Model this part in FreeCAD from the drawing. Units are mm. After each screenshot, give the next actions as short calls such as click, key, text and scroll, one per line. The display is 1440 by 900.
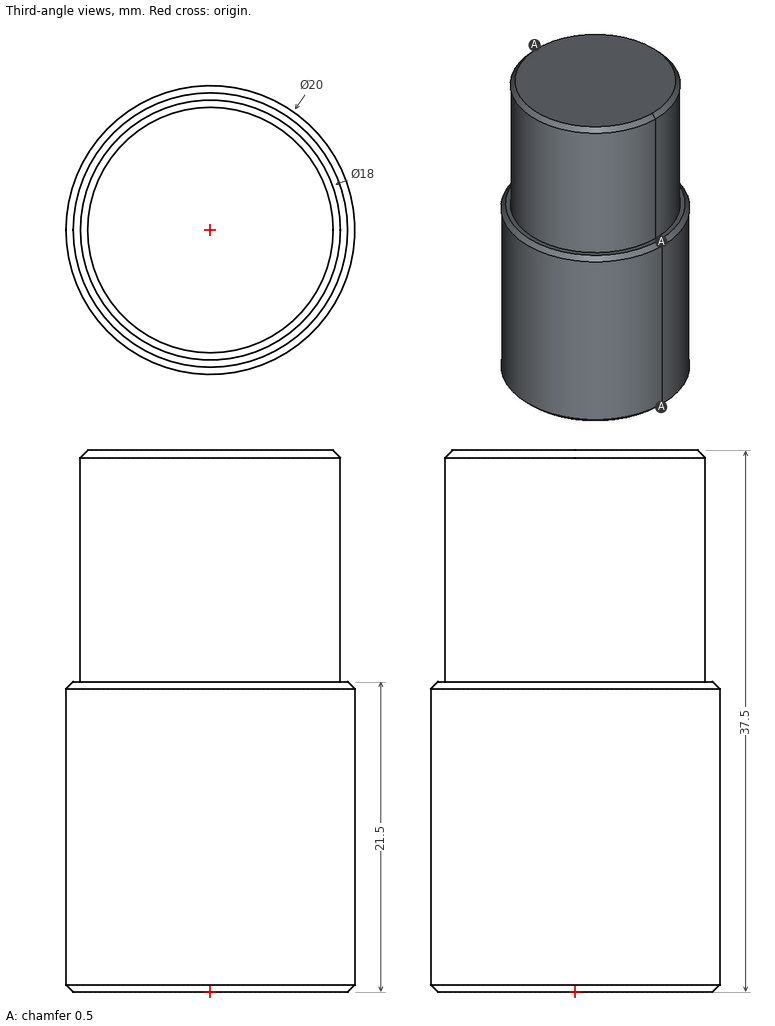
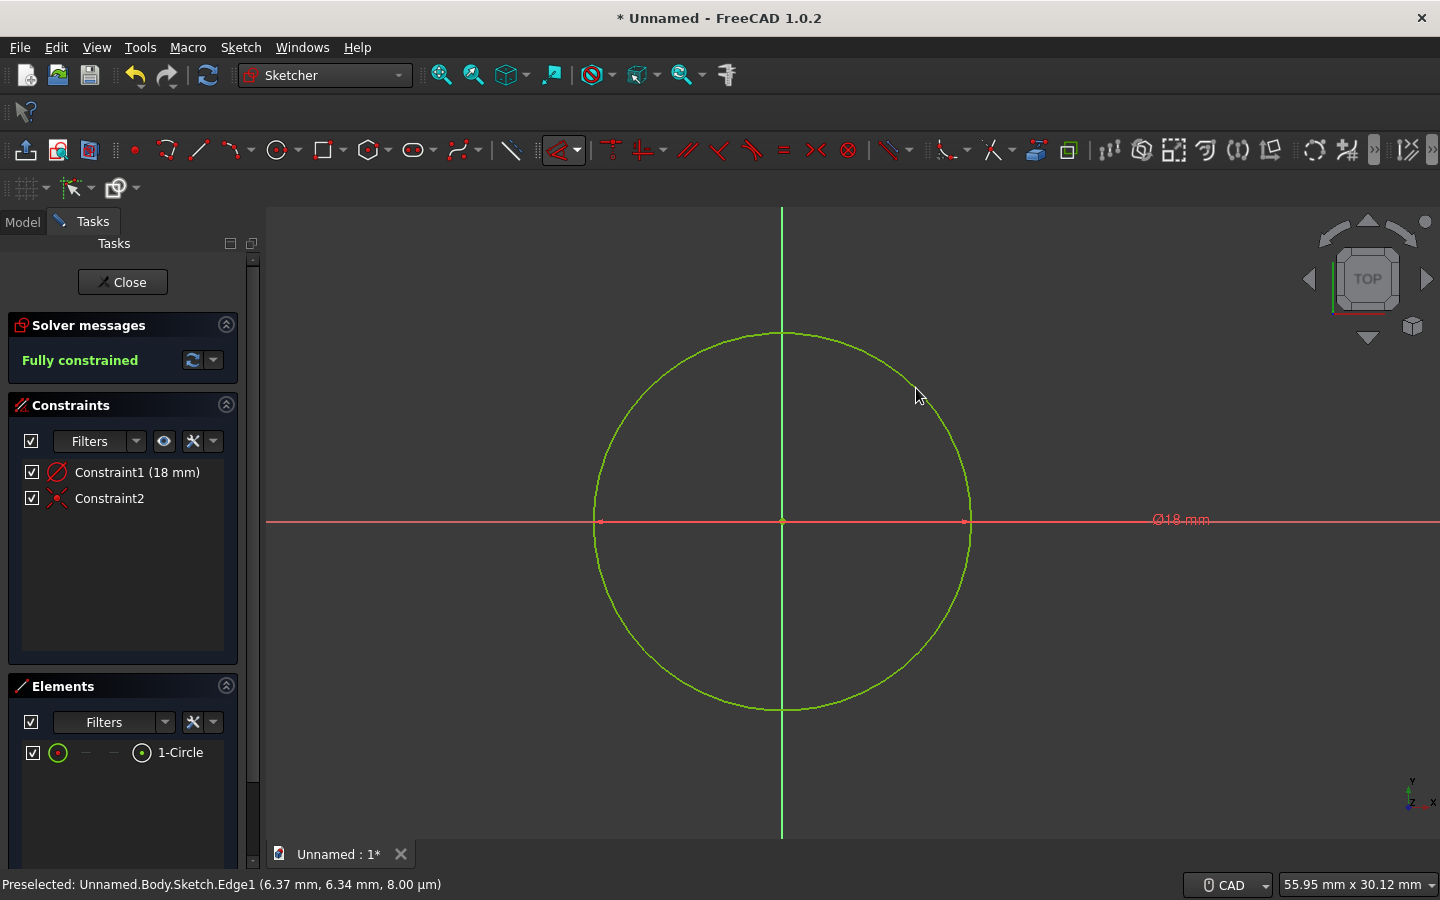
click(123, 282)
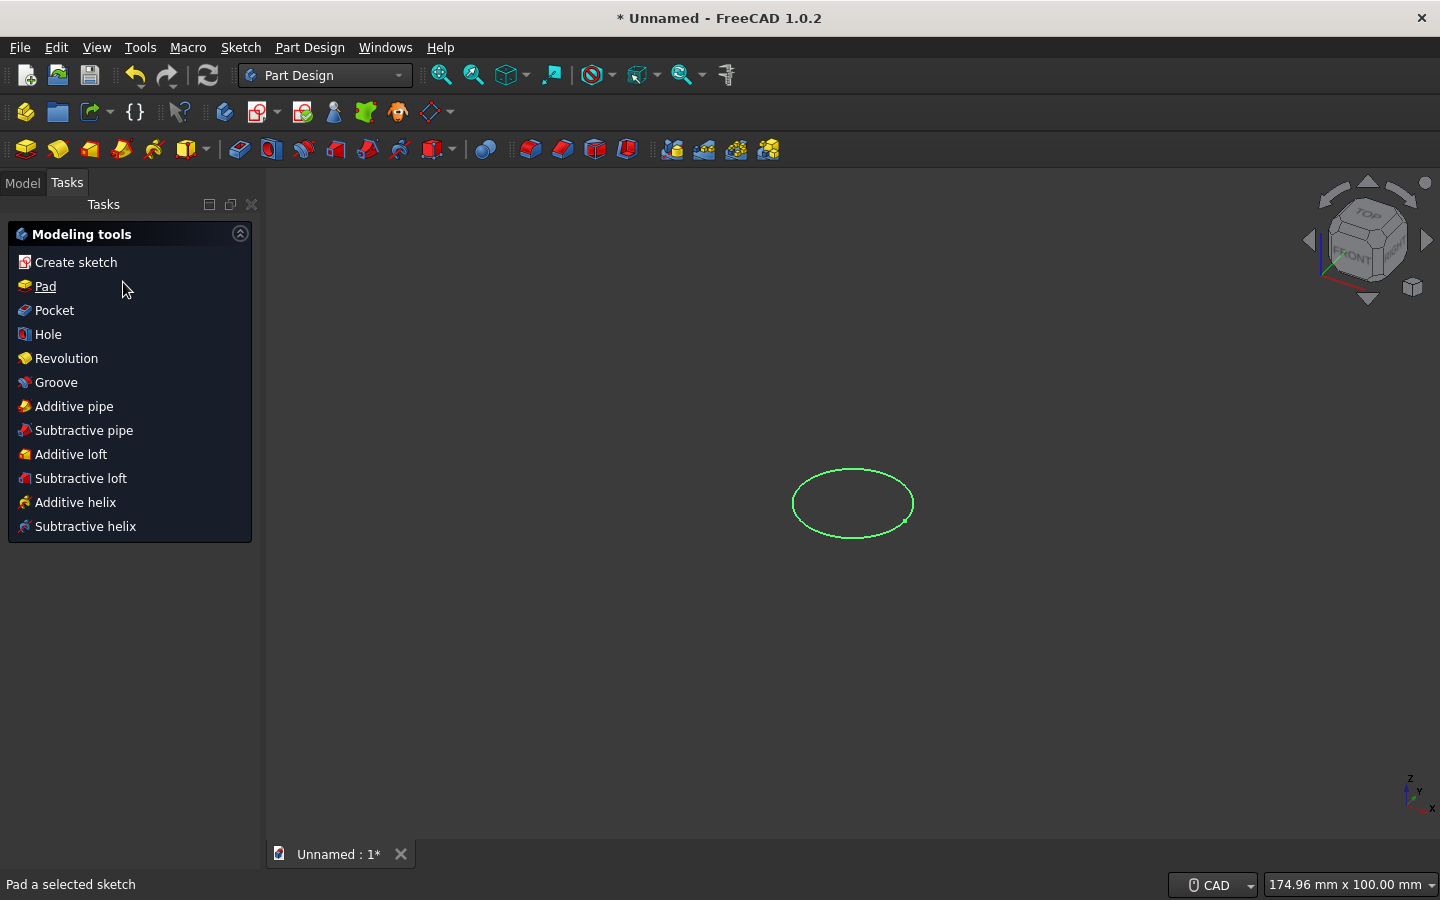
click(26, 150)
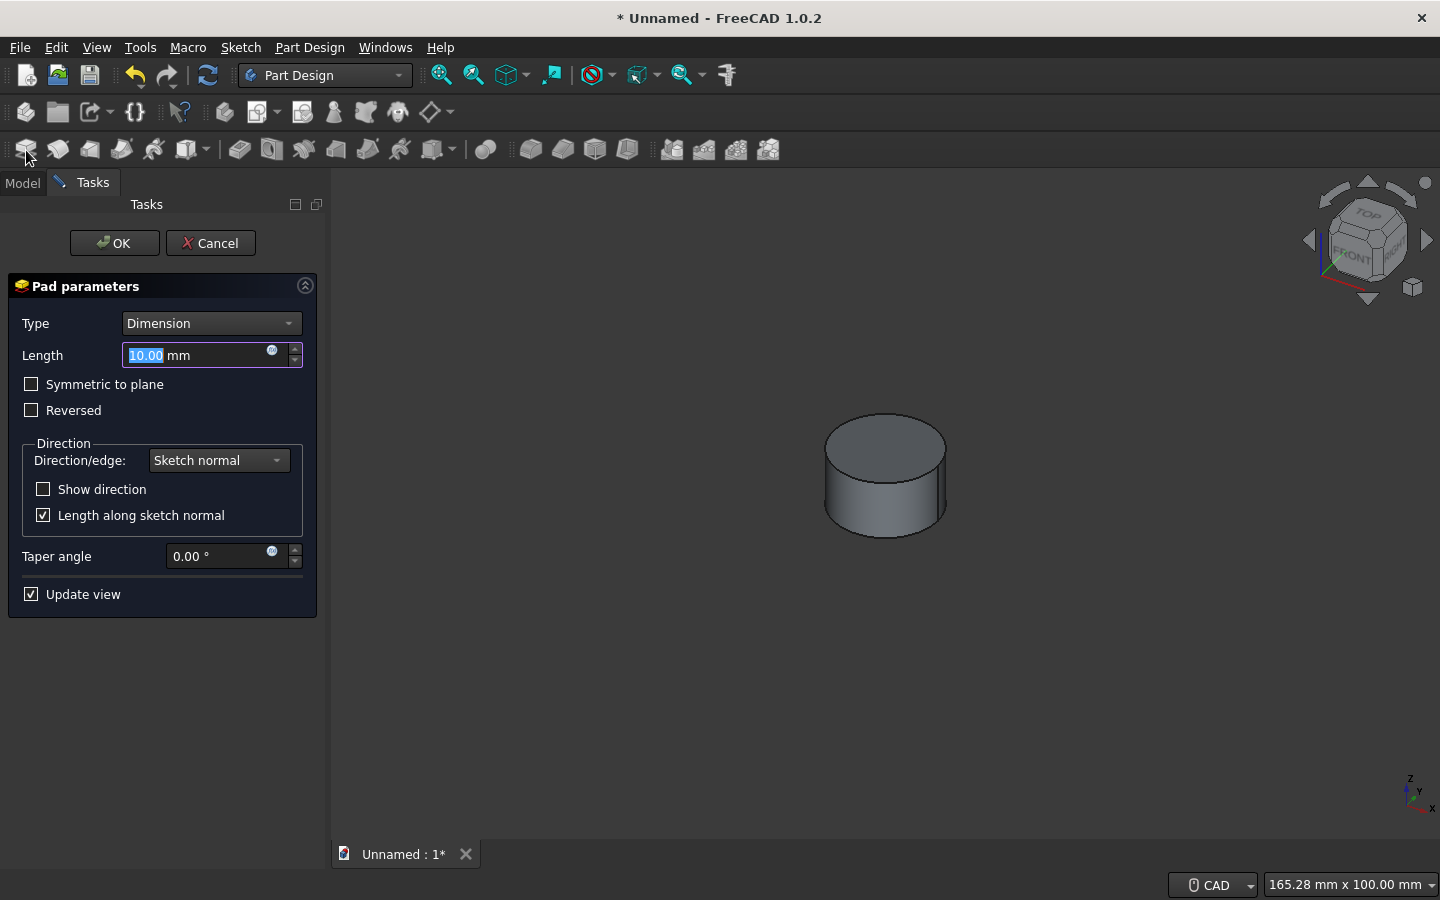
text(37.5)
key(Tab)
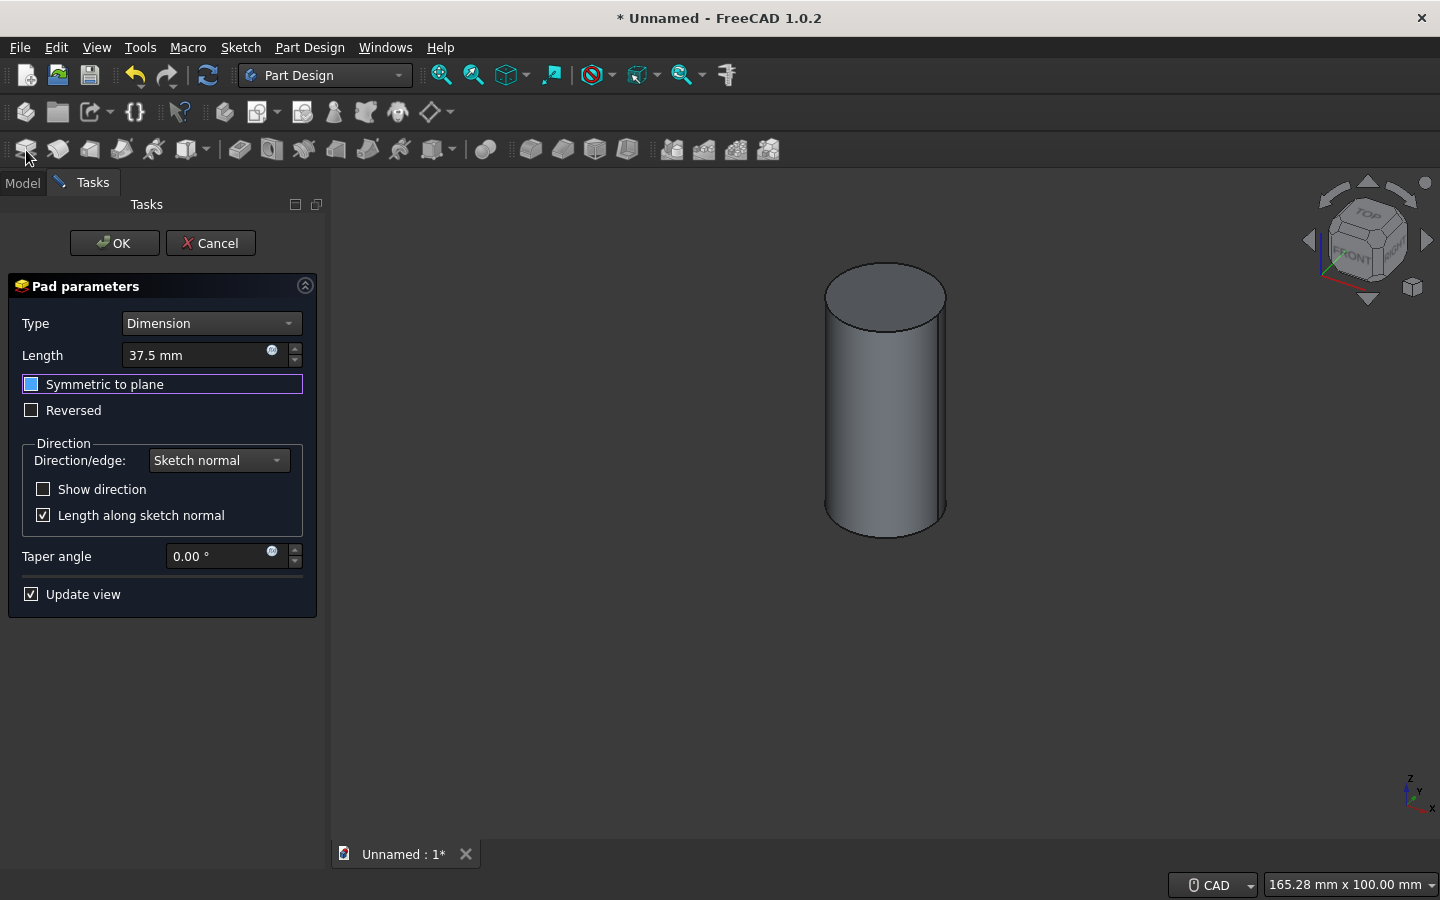
click(115, 243)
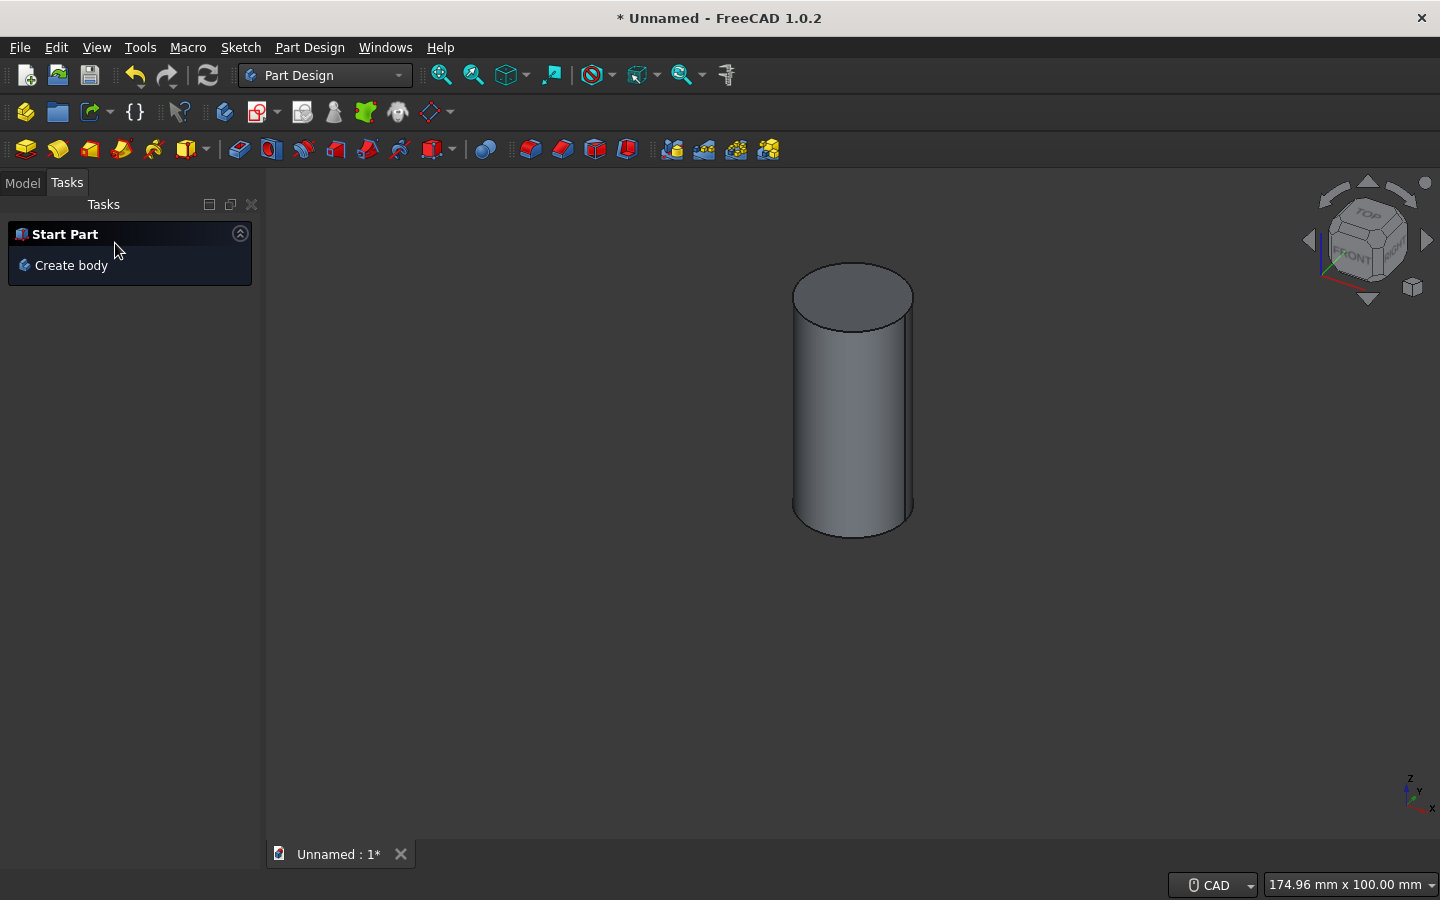
click(442, 76)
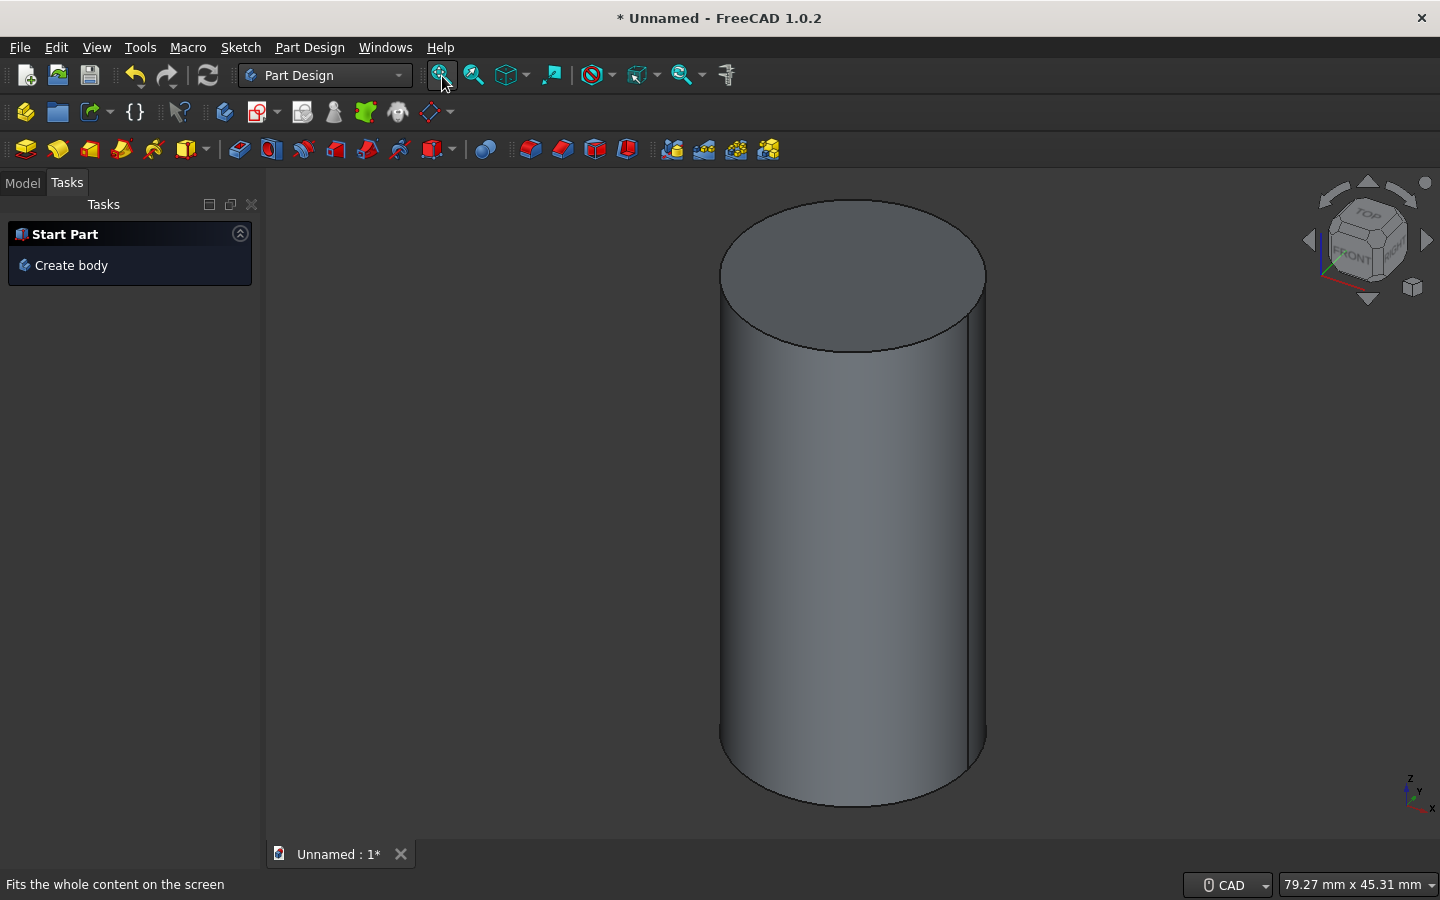
key(5)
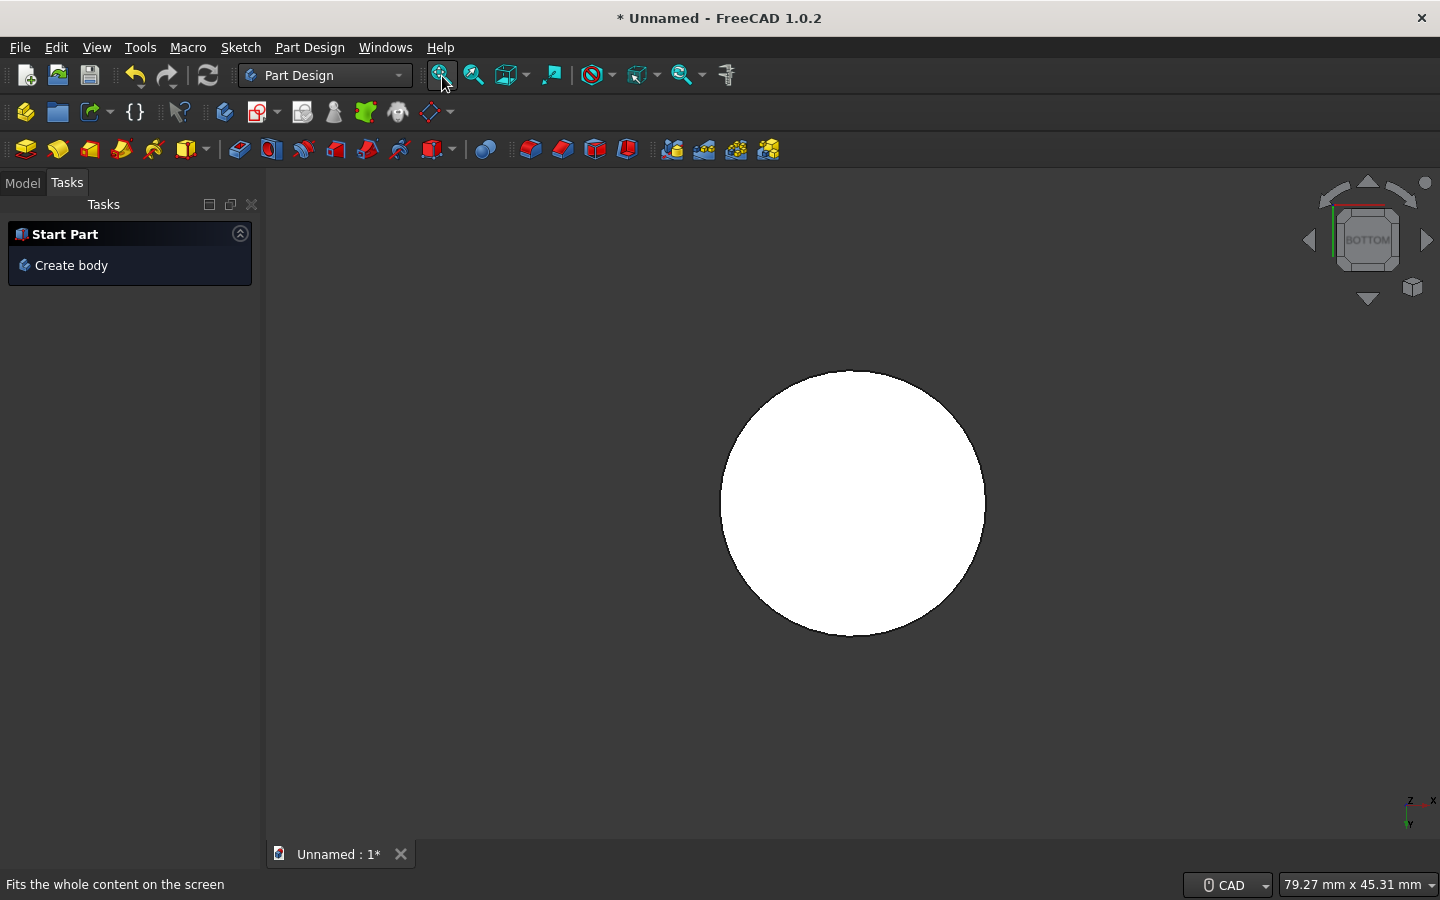
click(442, 76)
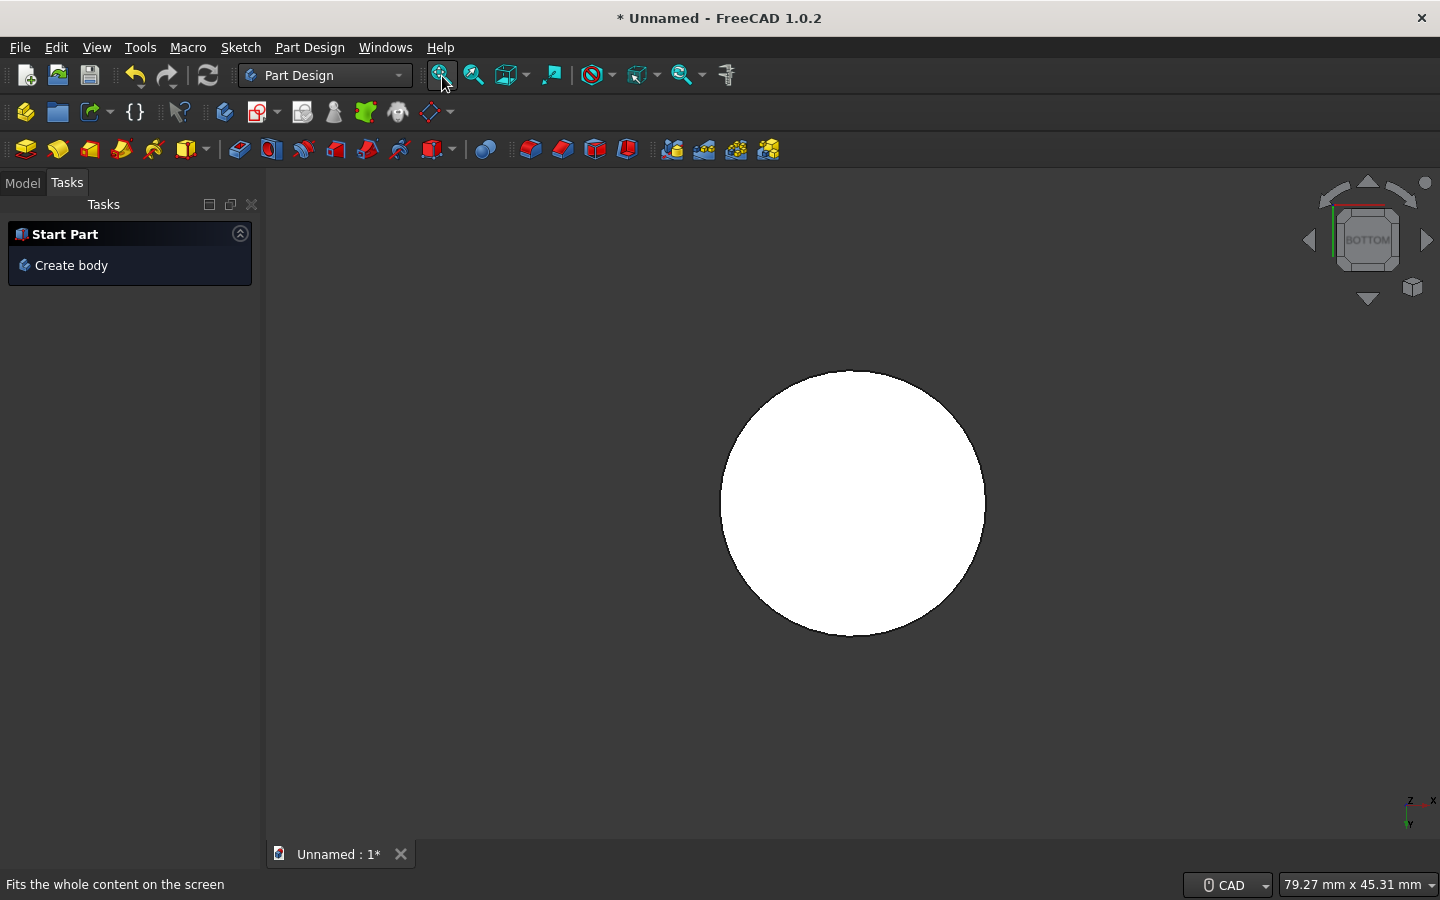
click(853, 502)